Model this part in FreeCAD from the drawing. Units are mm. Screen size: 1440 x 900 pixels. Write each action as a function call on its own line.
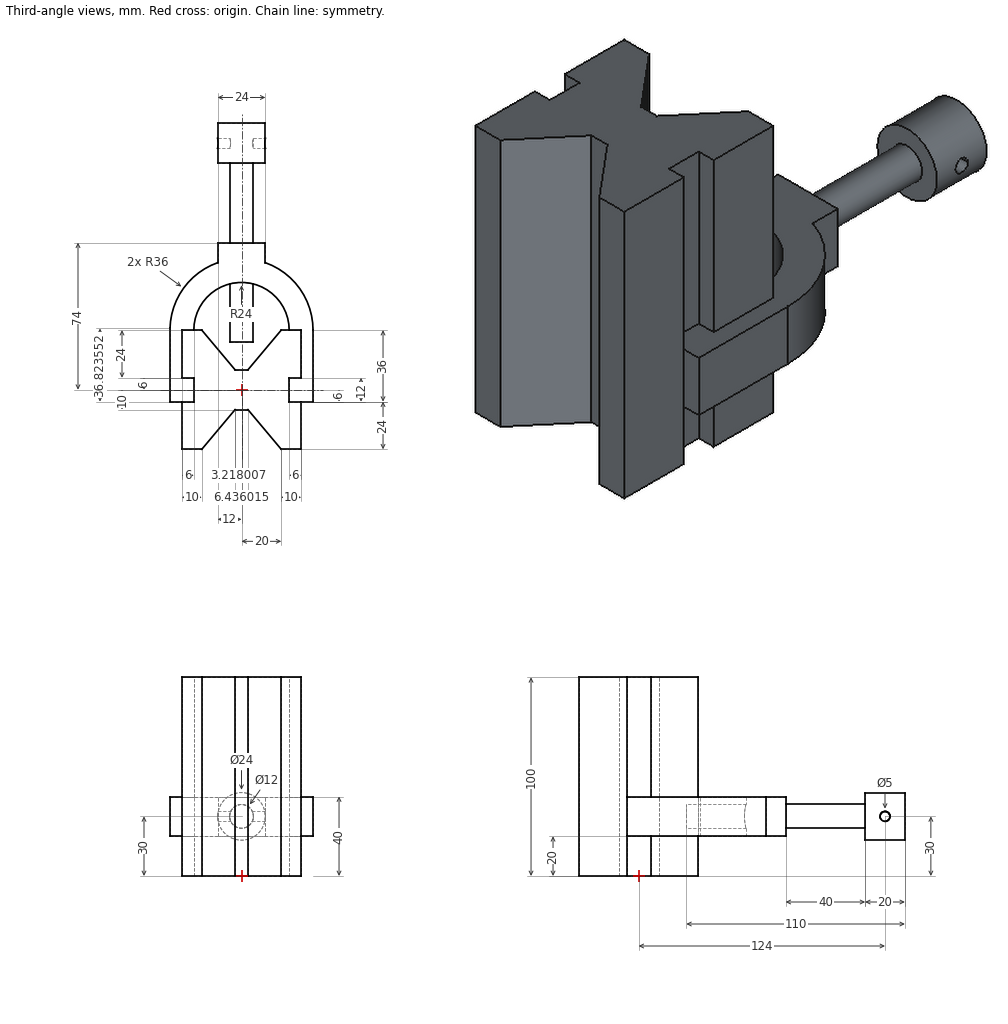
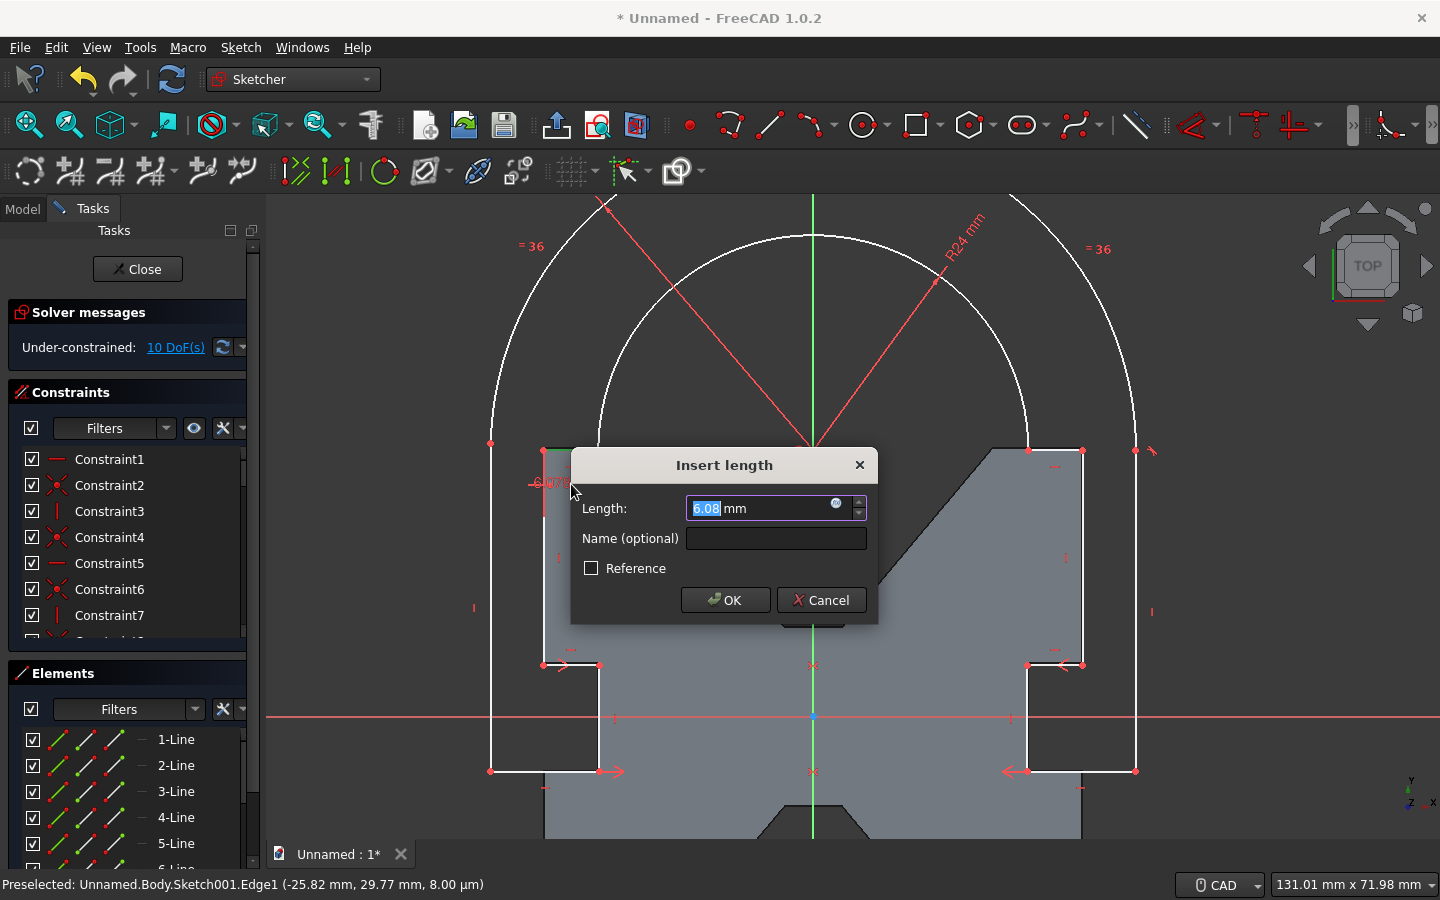
text(6)
key(Return)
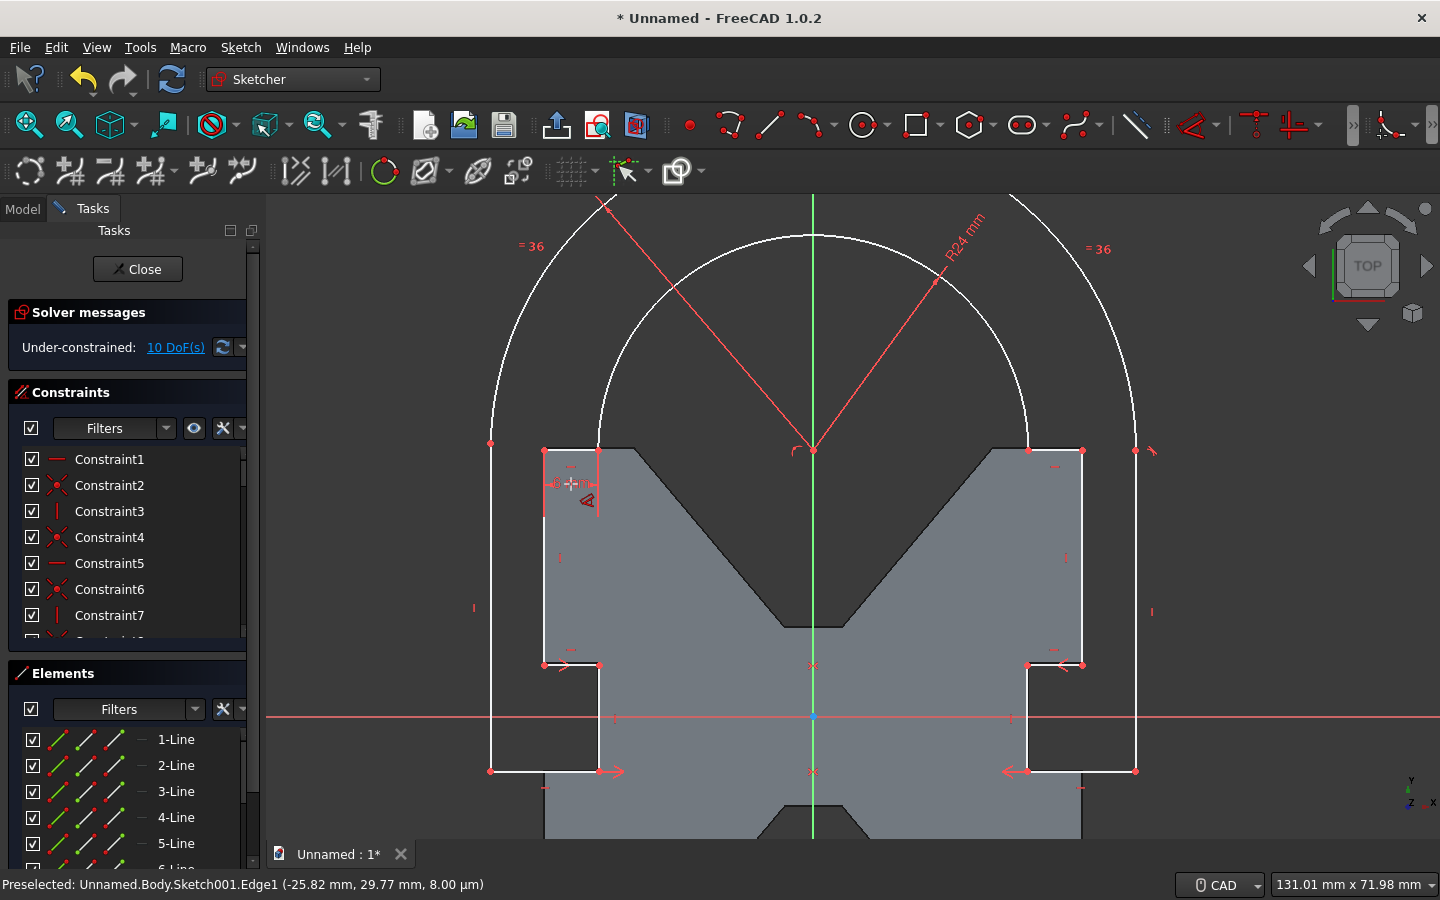
click(561, 665)
click(572, 699)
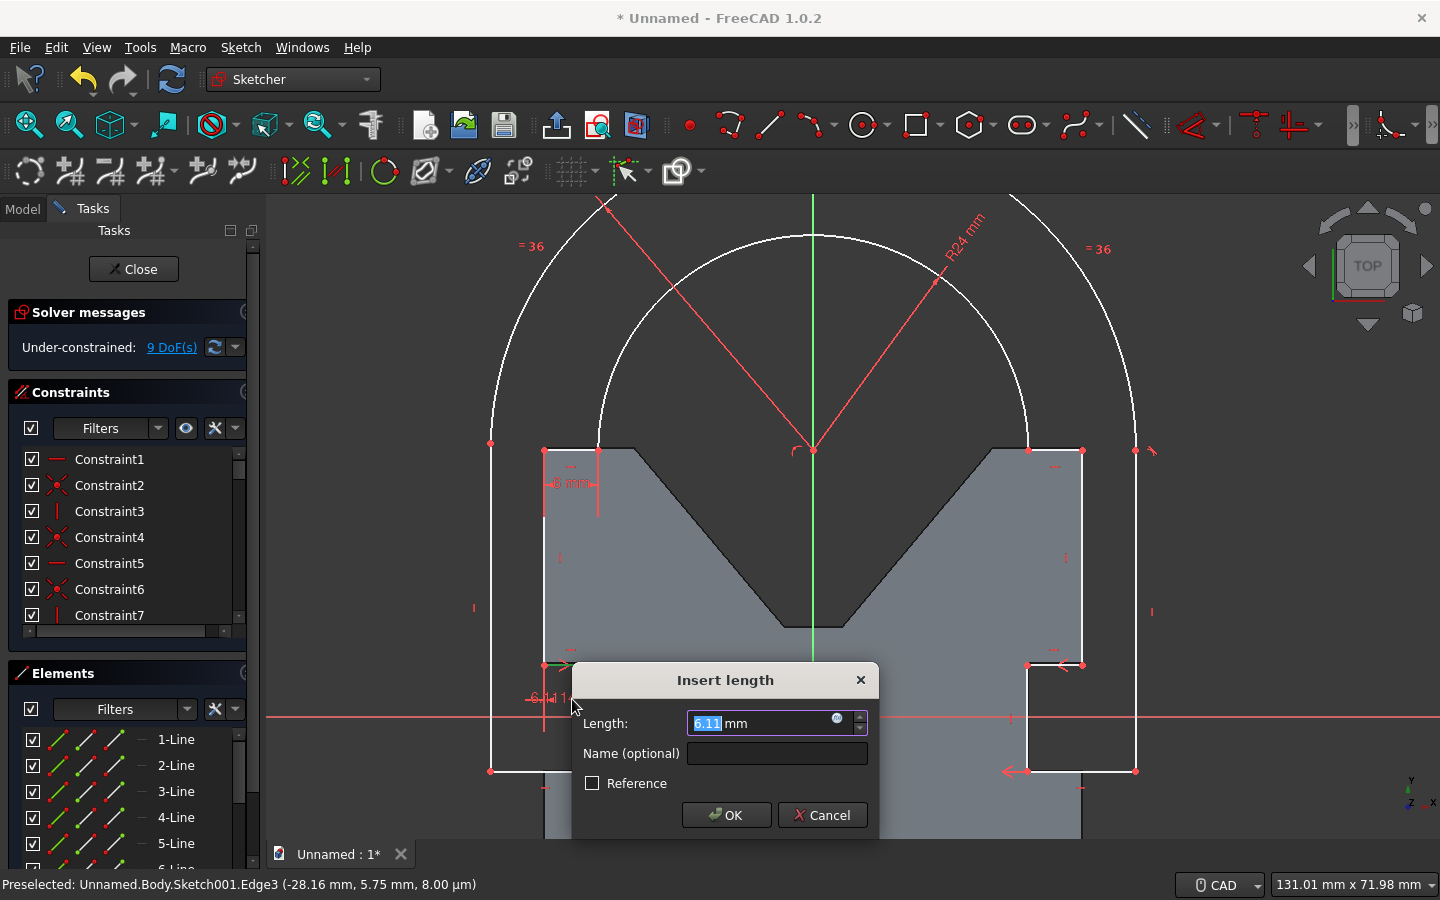
text(6)
key(Return)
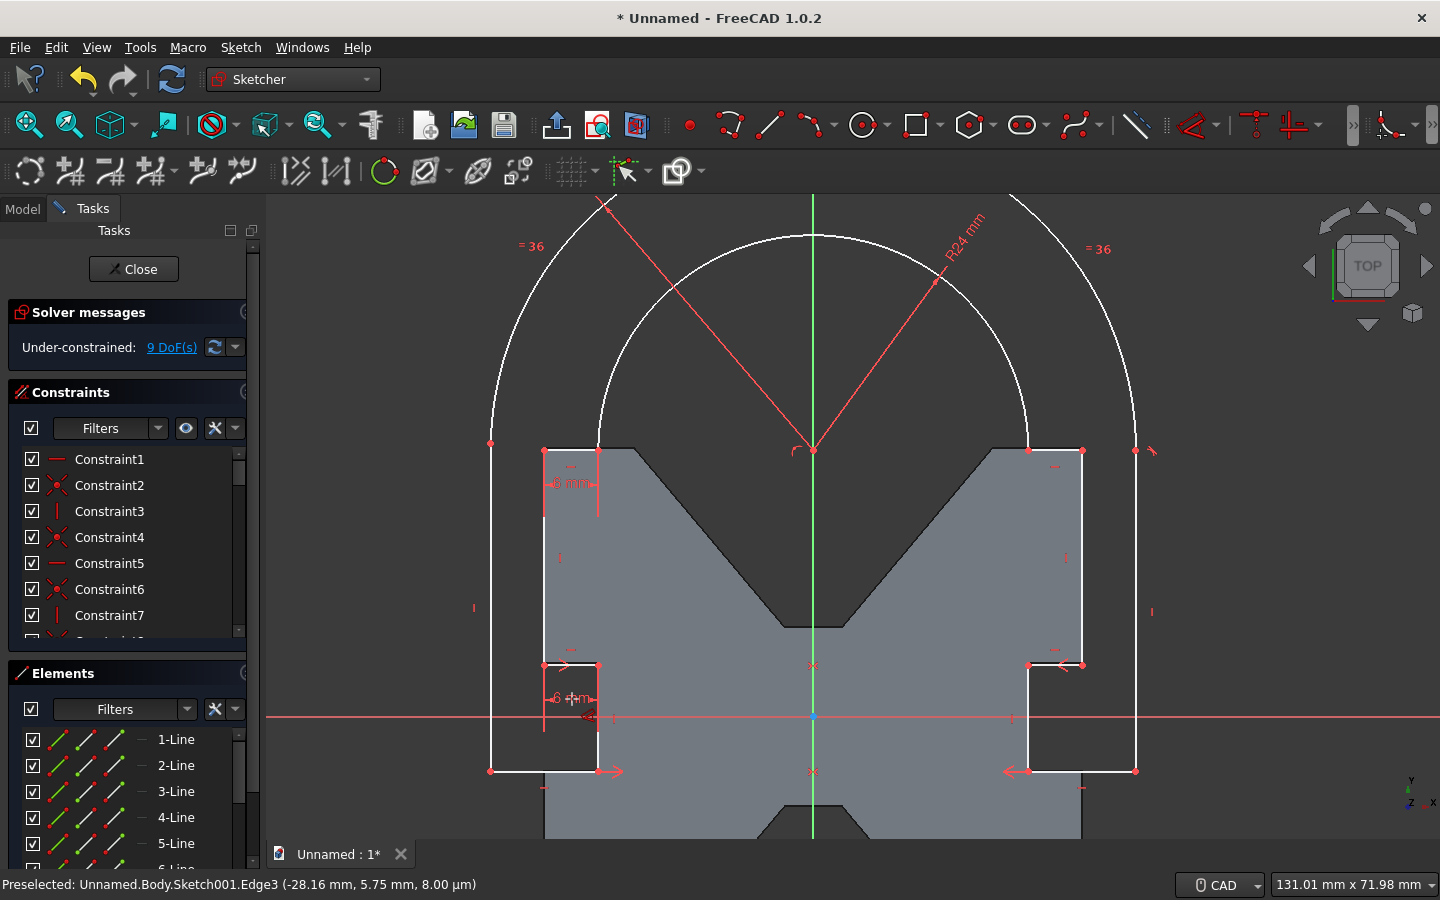
click(544, 515)
click(510, 558)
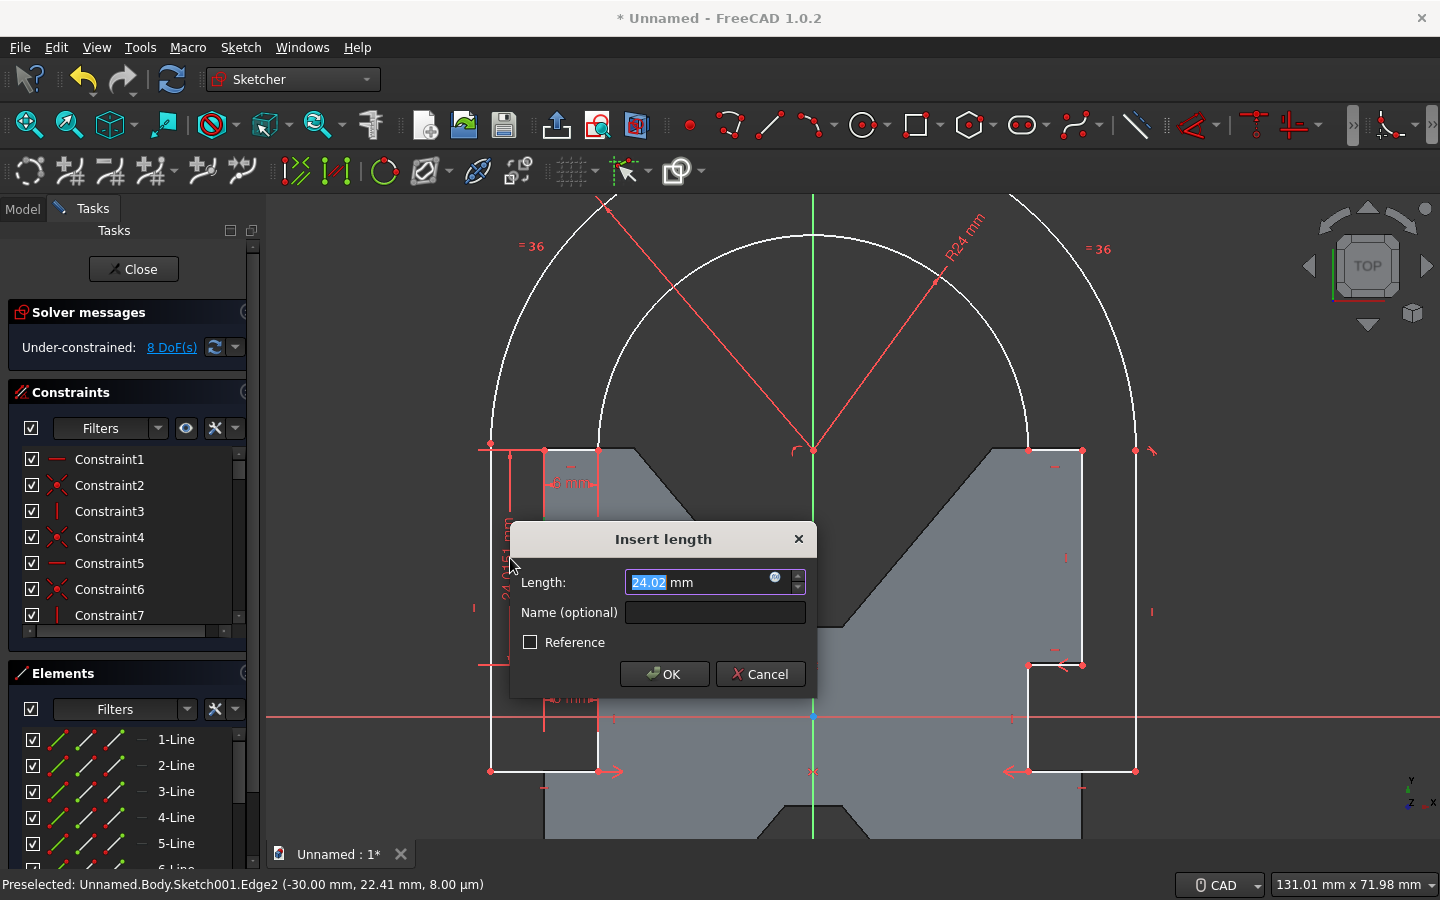
text(24)
key(Return)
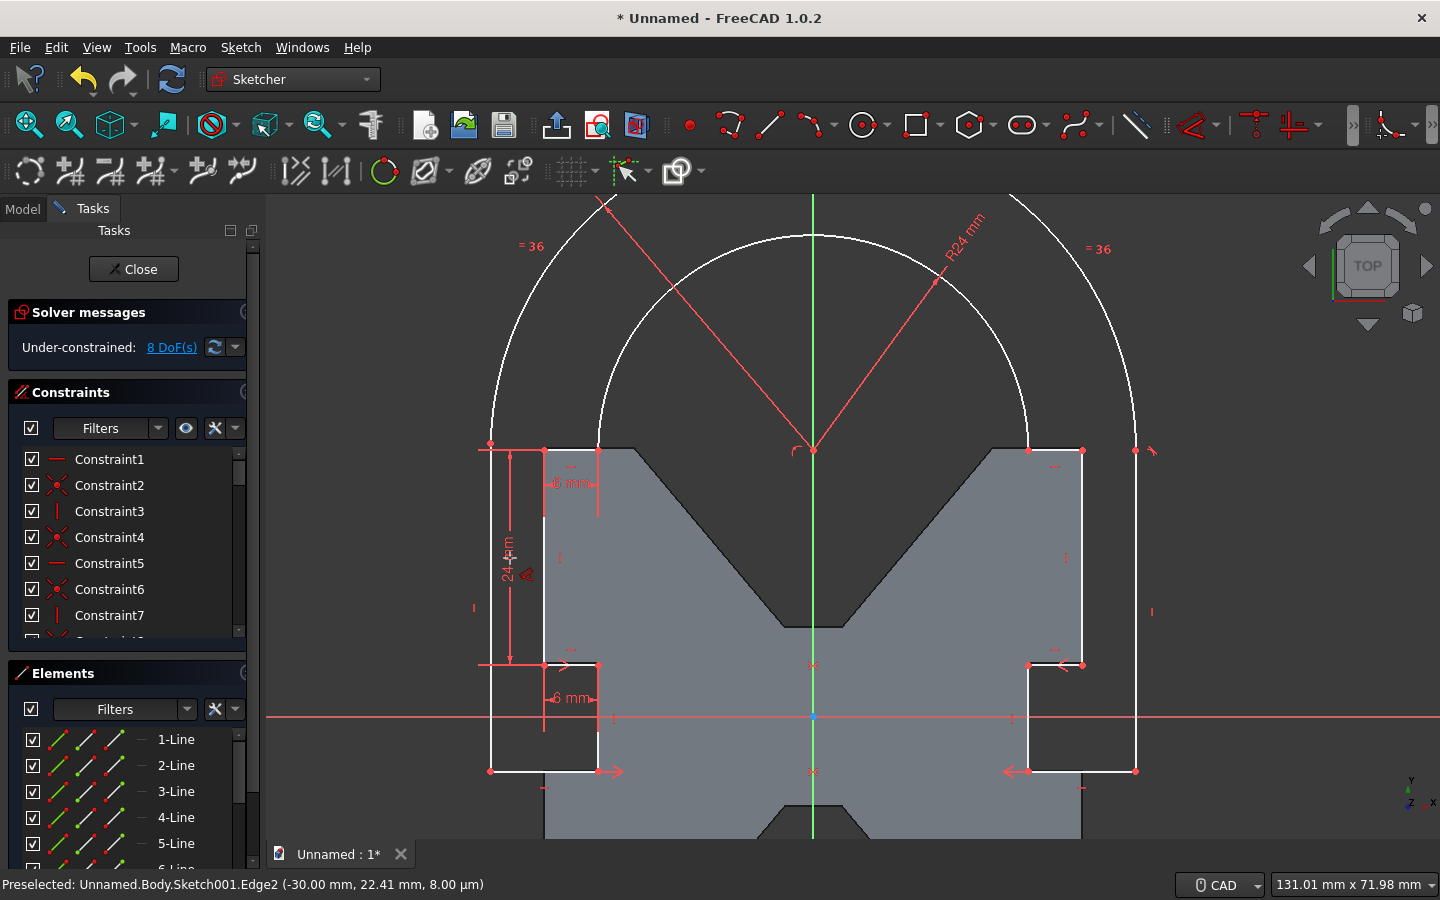
click(598, 697)
click(564, 743)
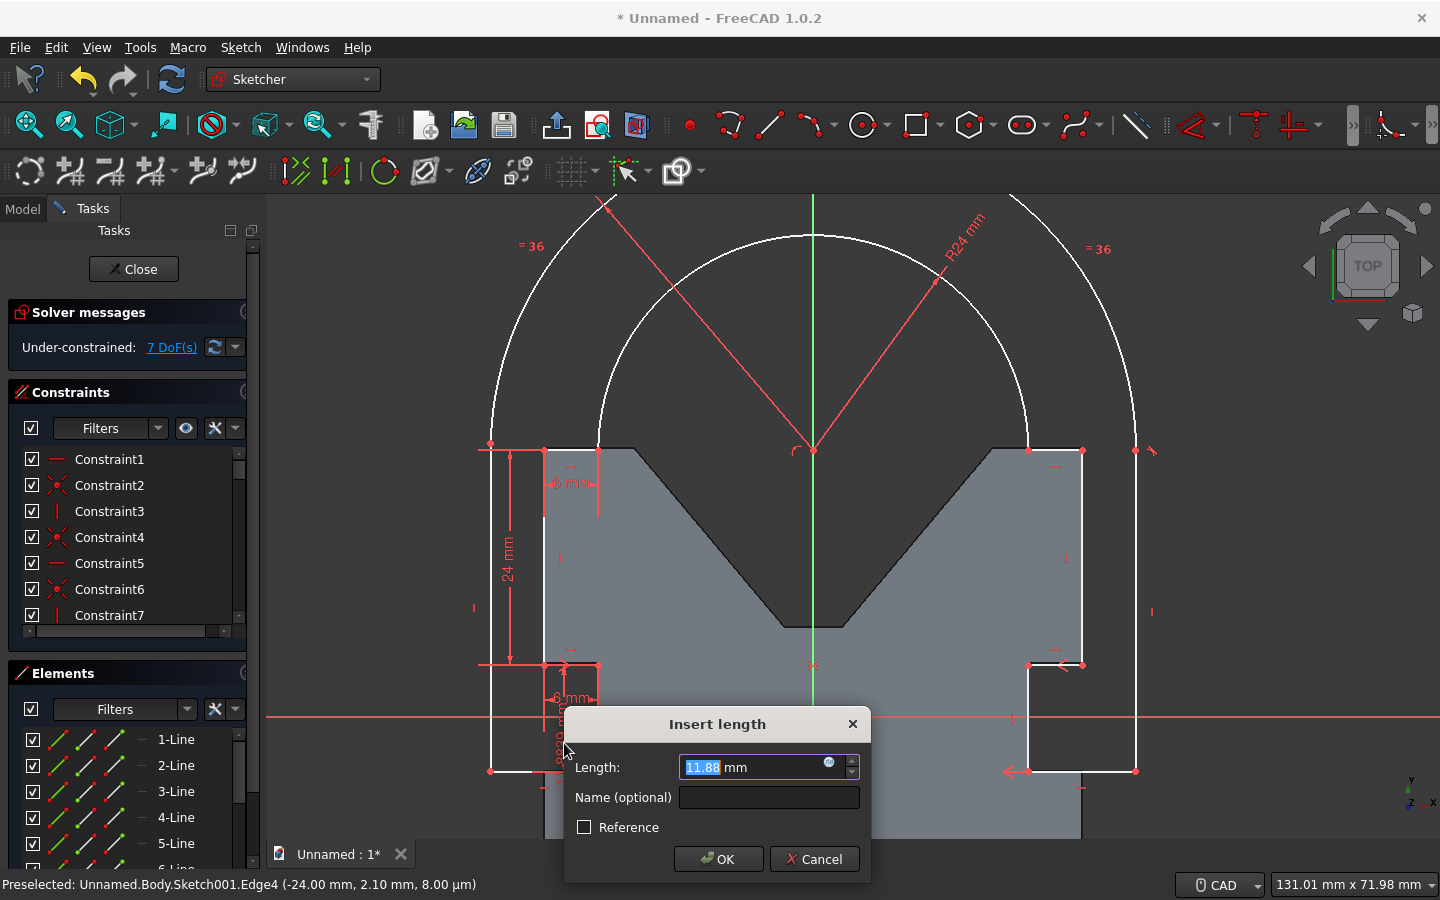
text(12)
key(Return)